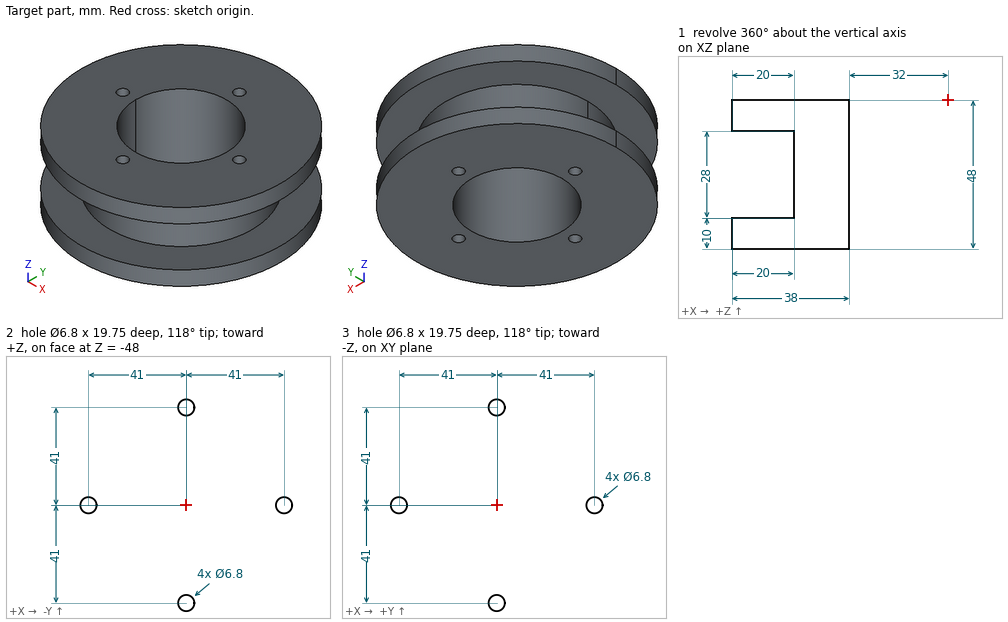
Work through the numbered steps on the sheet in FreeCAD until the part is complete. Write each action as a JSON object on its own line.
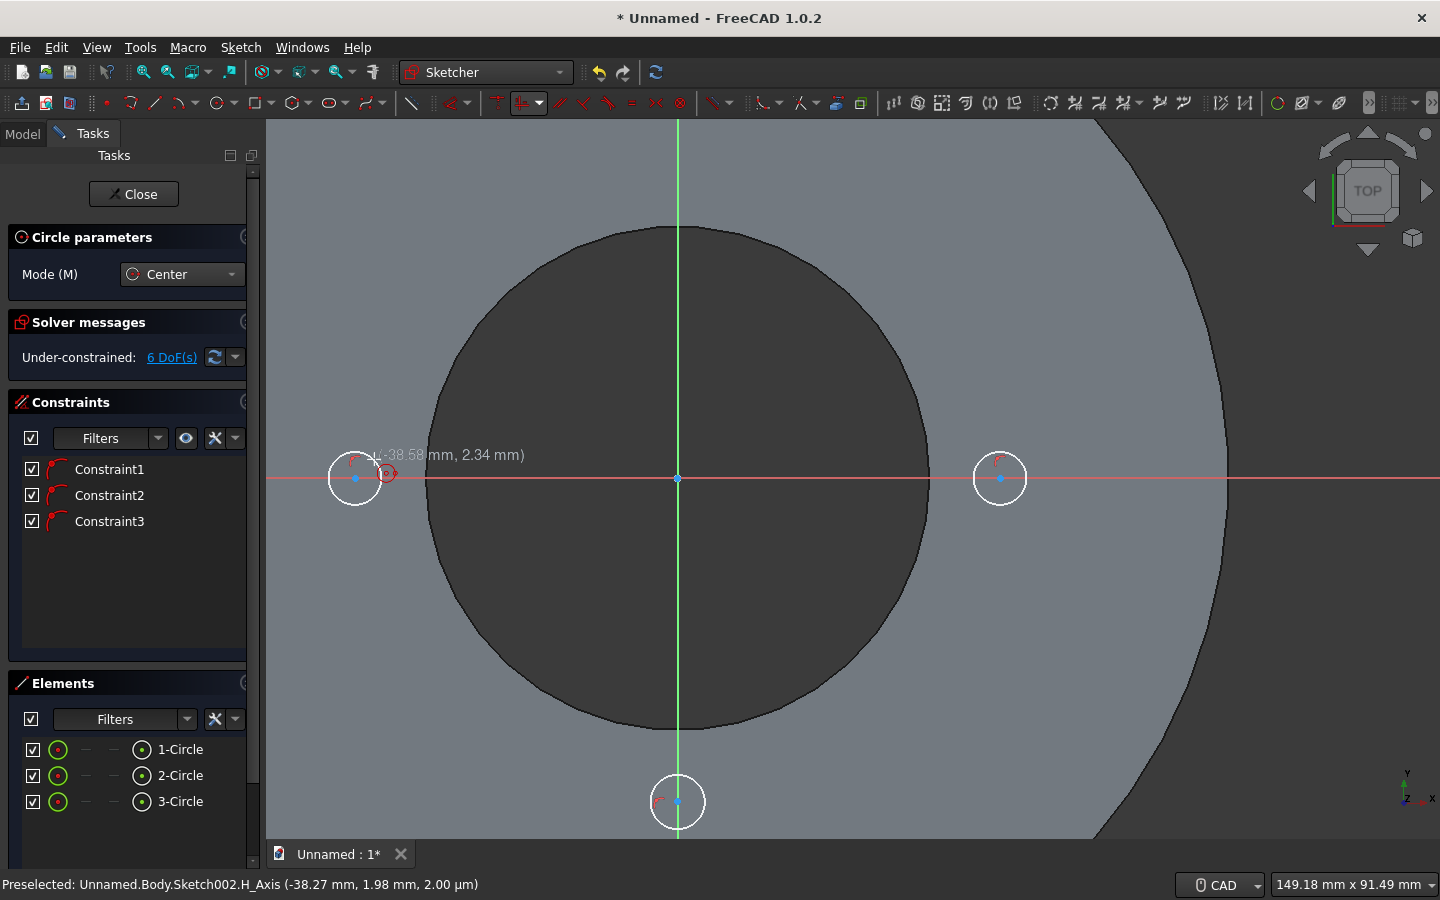
{"action": "left_click", "coordinate": [678, 156]}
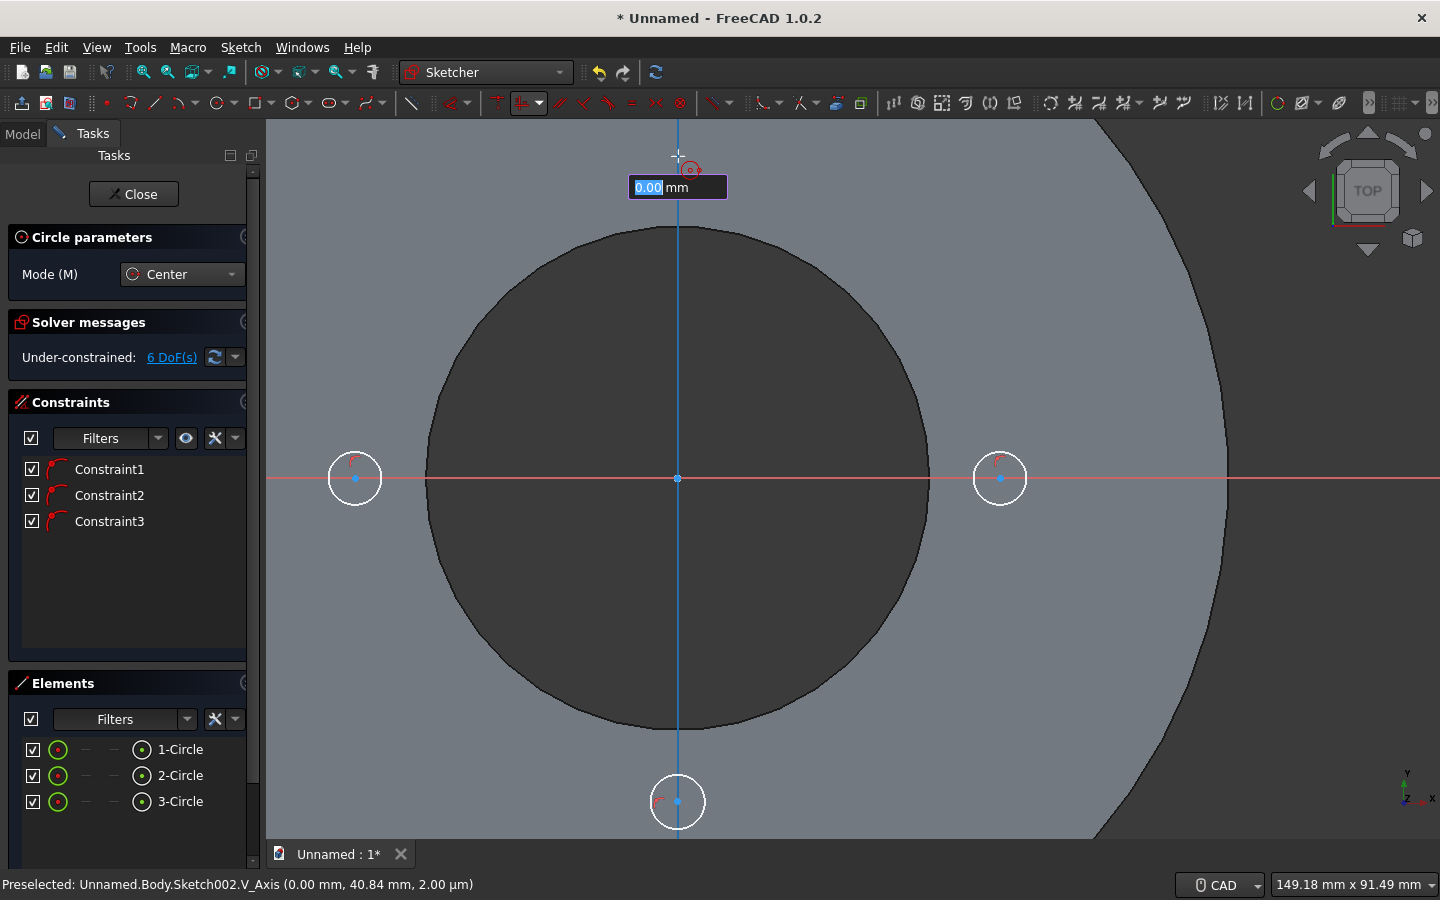
{"action": "scroll", "coordinate": [1002, 480], "scroll_direction": "down", "scroll_amount": 2}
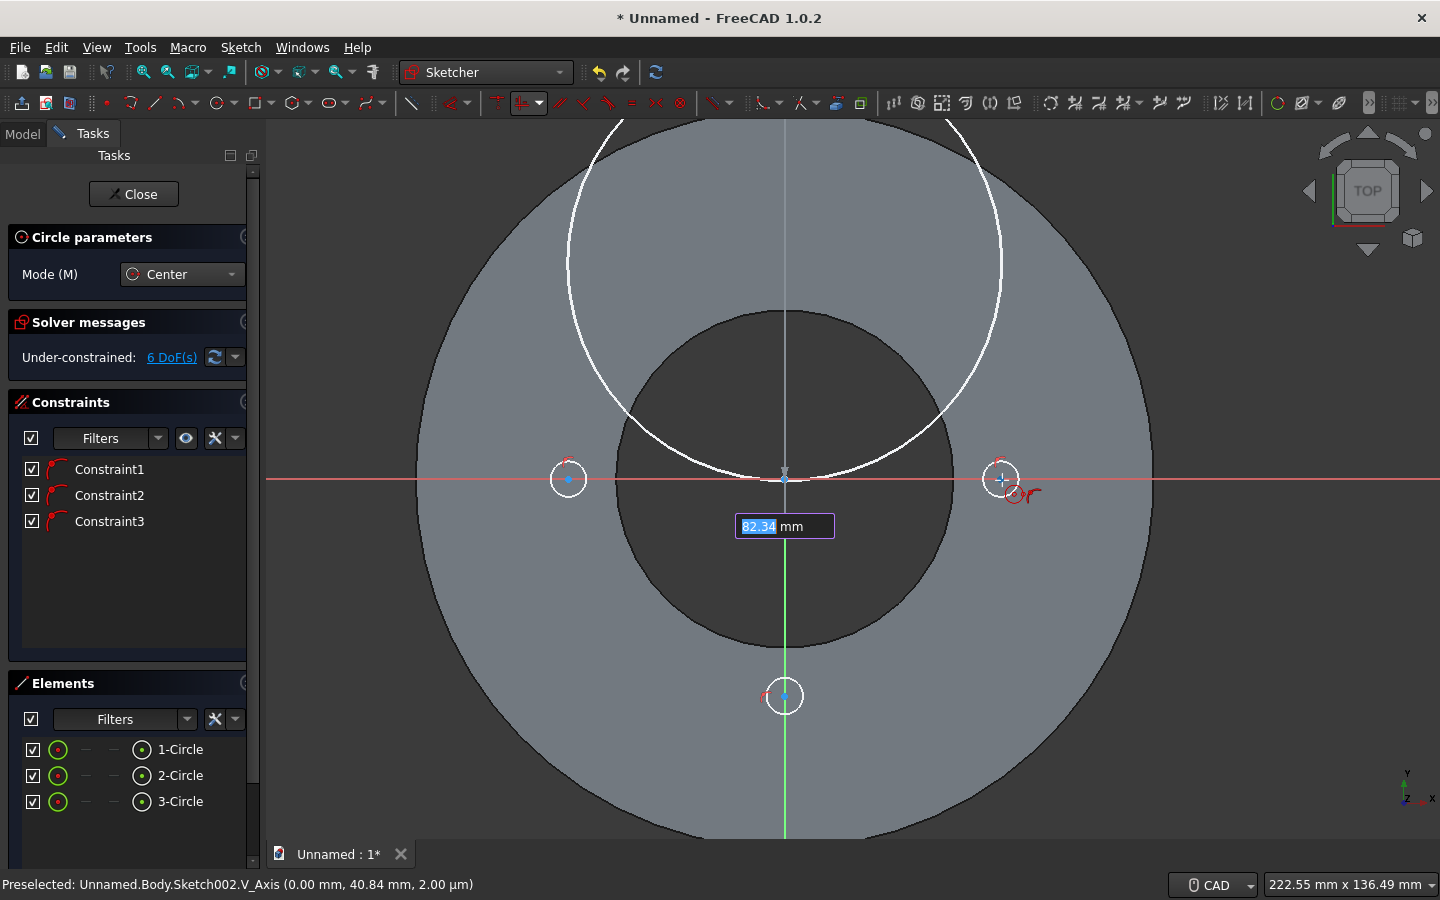
{"action": "scroll", "coordinate": [797, 250], "scroll_direction": "up", "scroll_amount": 2}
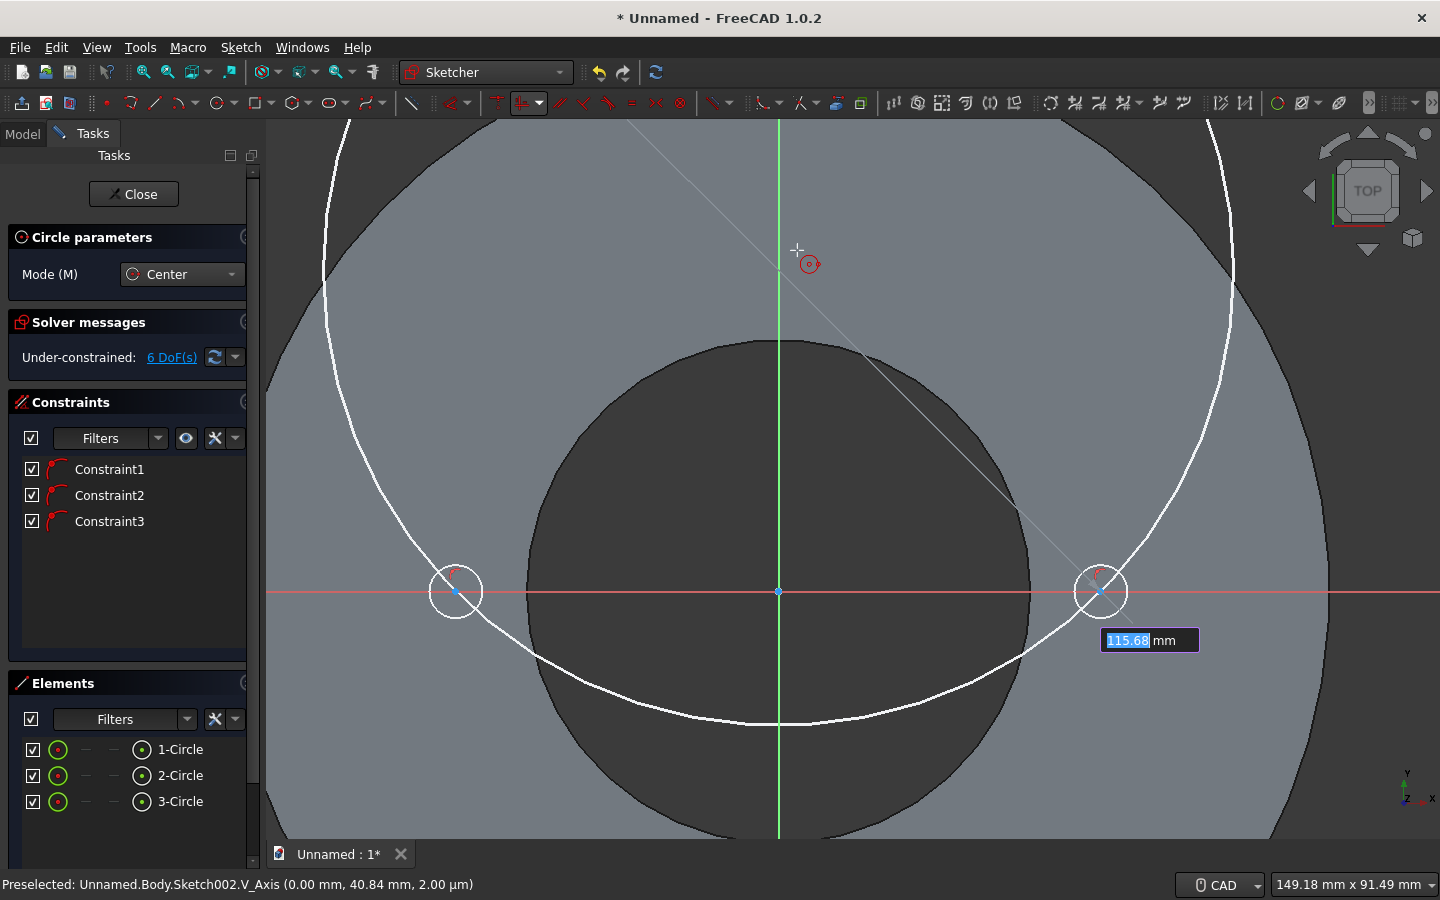
{"action": "left_click", "coordinate": [797, 250]}
{"action": "key", "text": "Escape"}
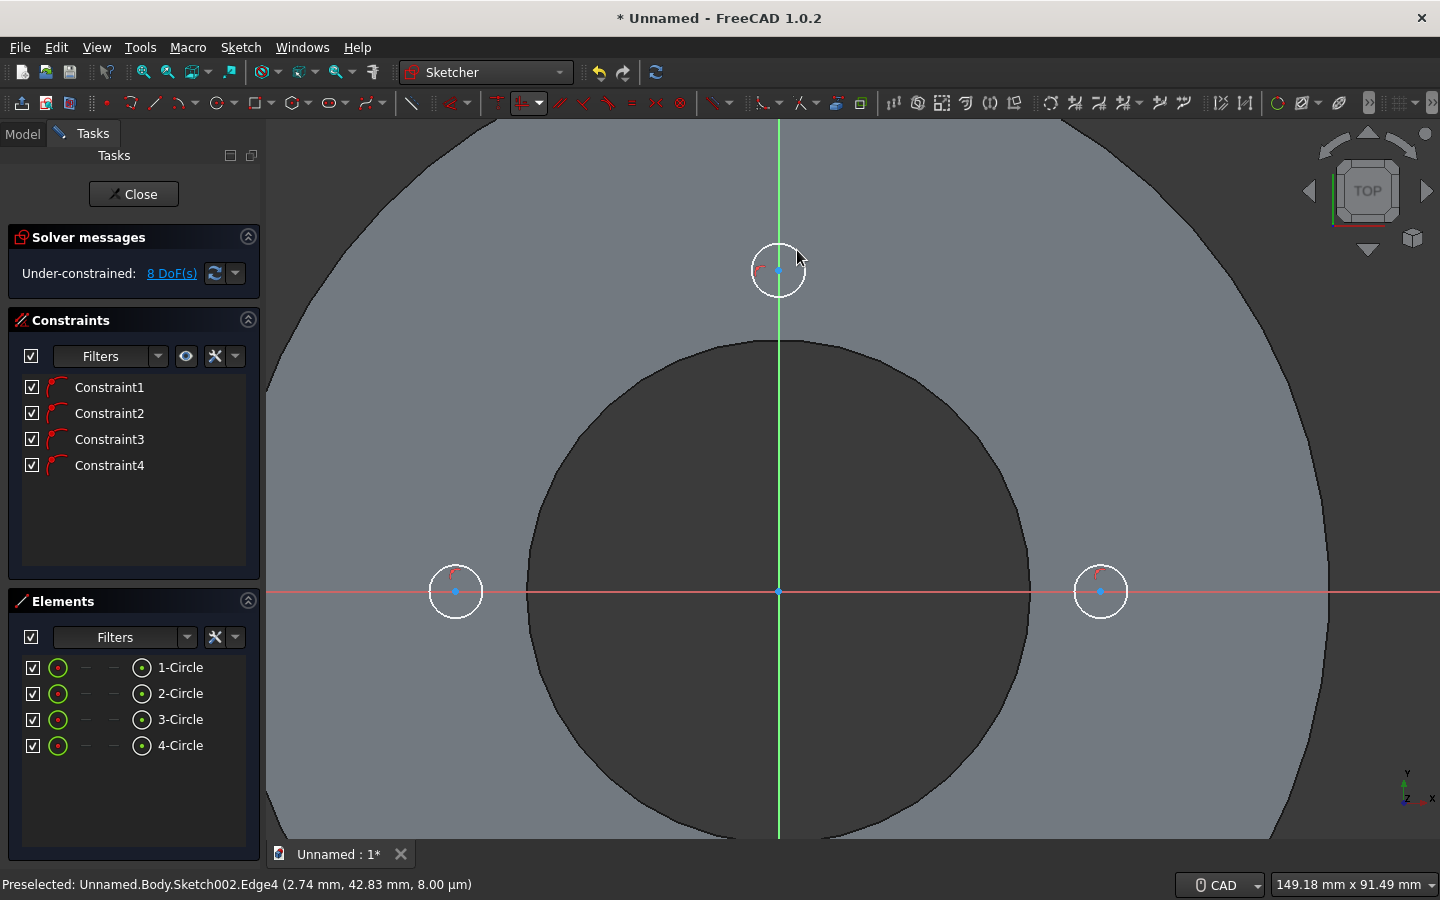
{"action": "left_click", "coordinate": [1120, 573]}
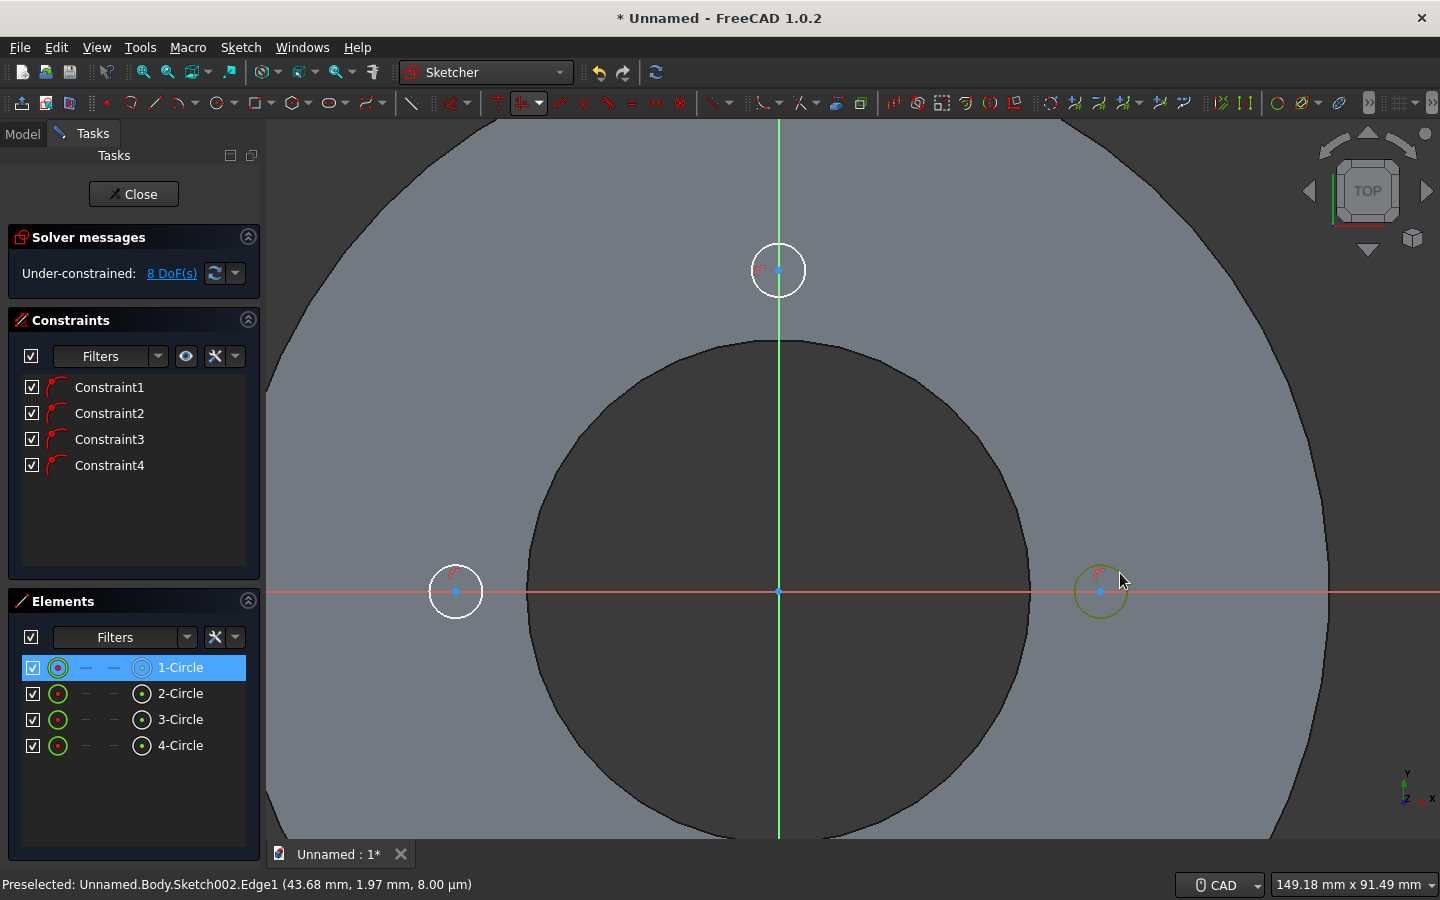
{"action": "scroll", "coordinate": [797, 250], "scroll_direction": "down", "scroll_amount": 2}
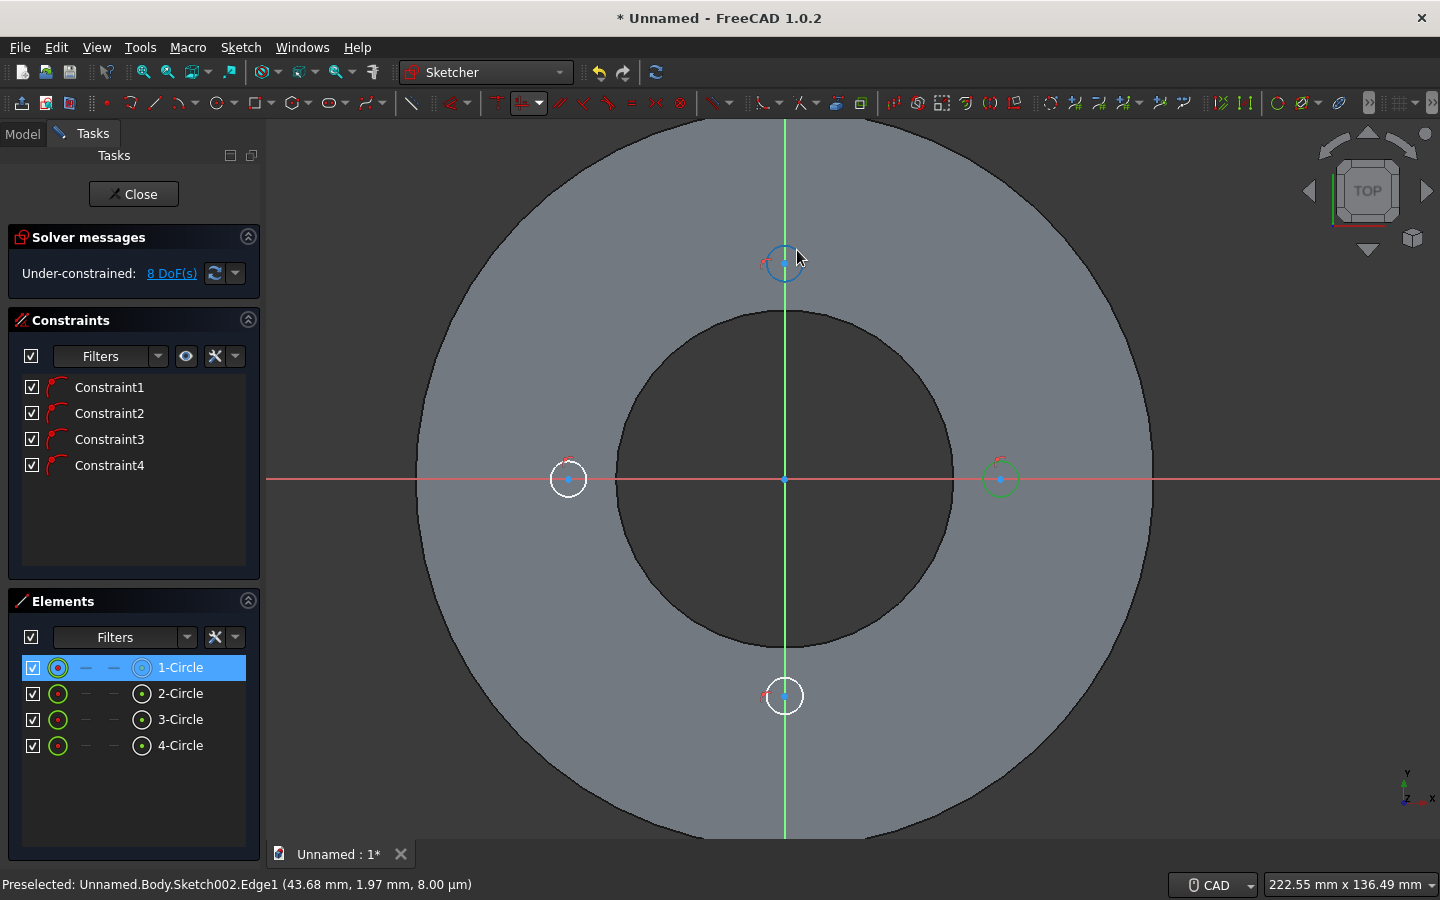
{"action": "left_click", "coordinate": [798, 683]}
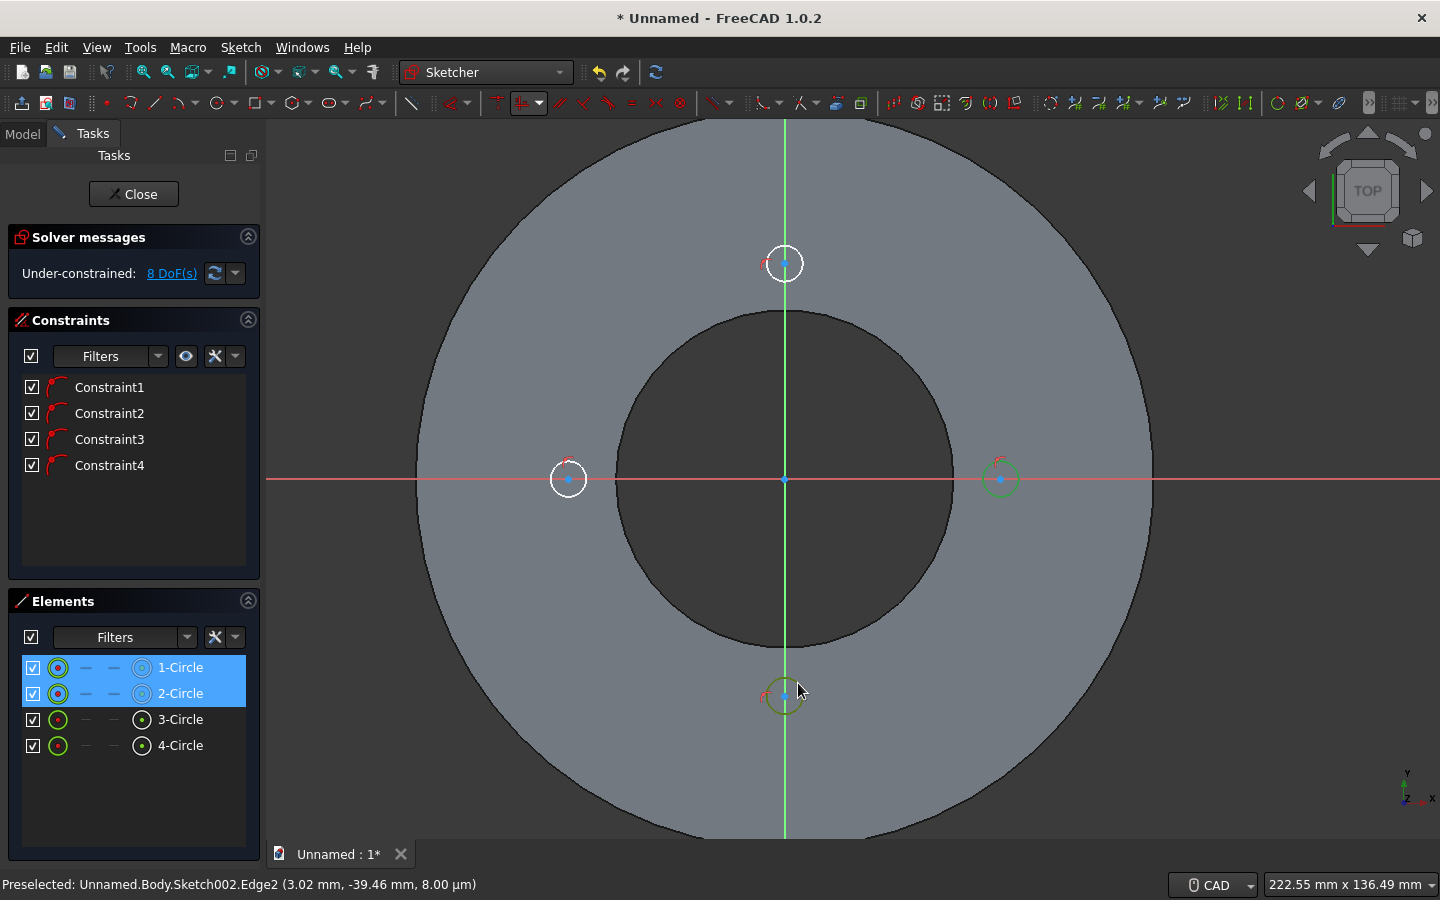
{"action": "left_click", "coordinate": [581, 467]}